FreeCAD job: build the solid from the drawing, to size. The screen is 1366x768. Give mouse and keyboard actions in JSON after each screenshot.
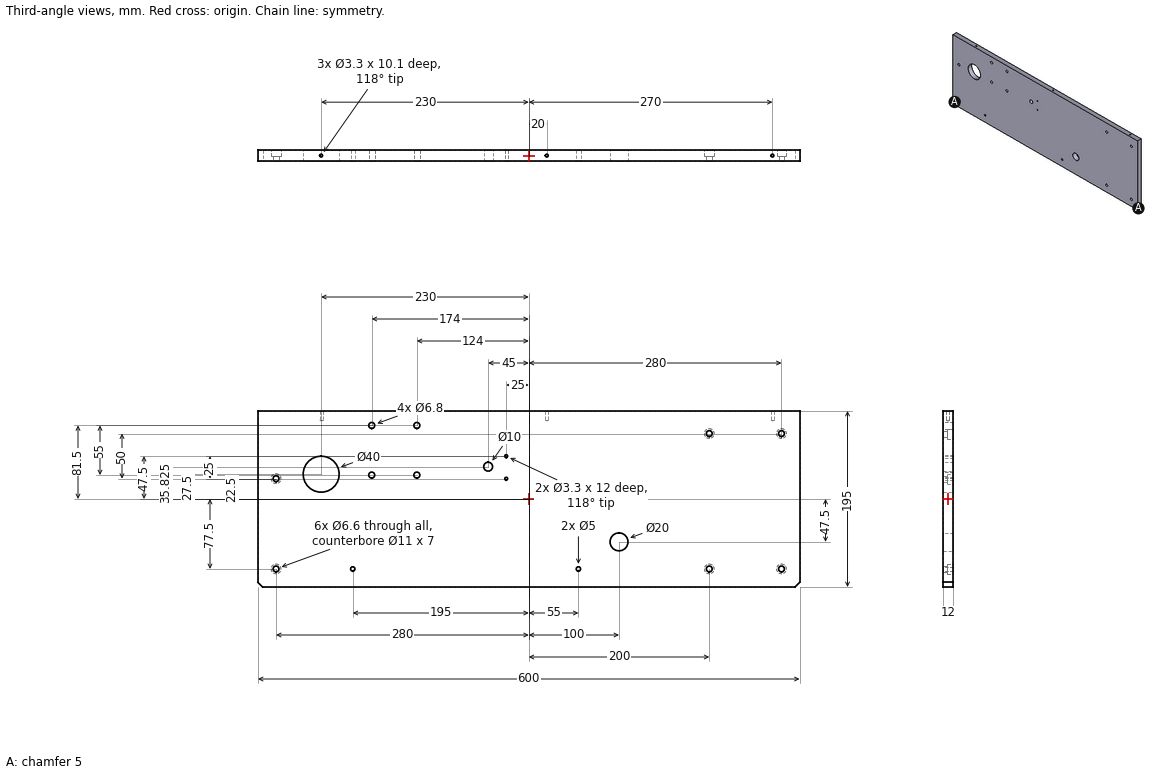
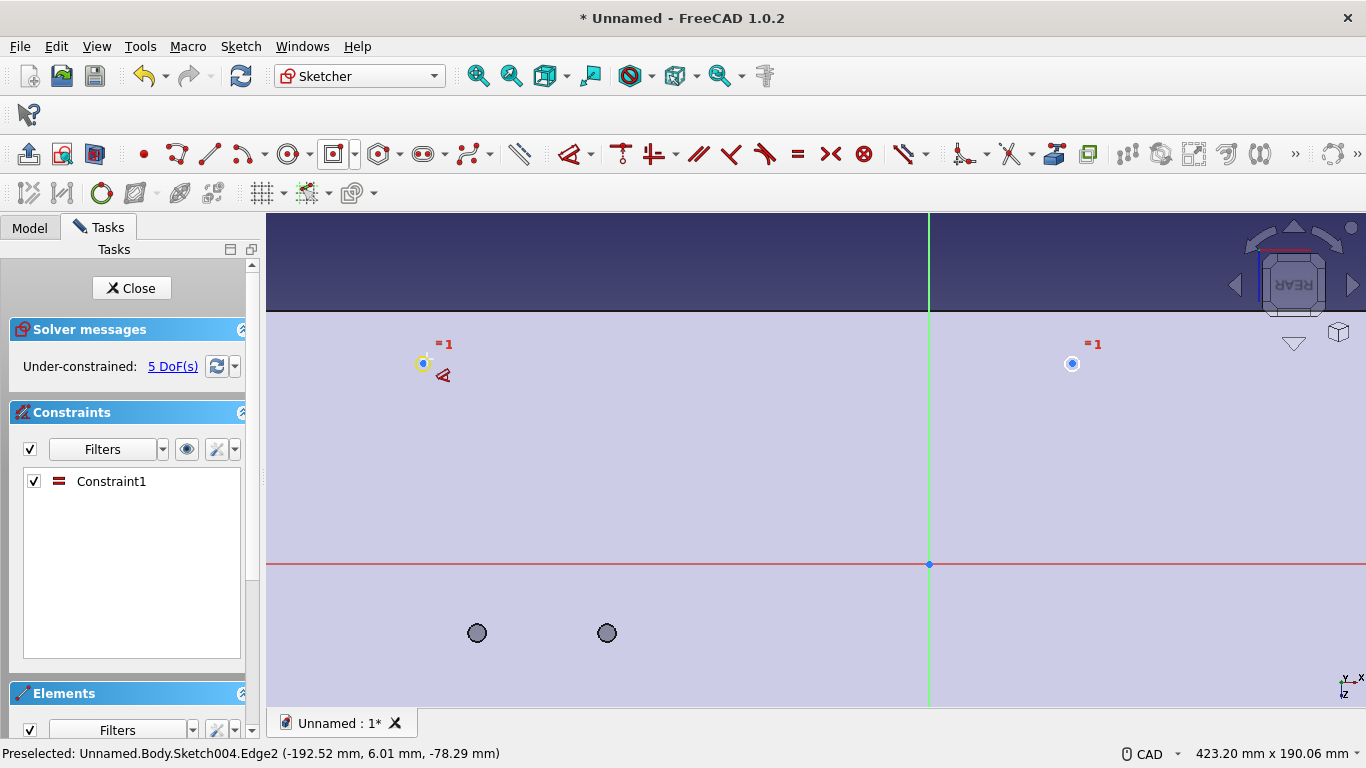
{"action": "scroll", "coordinate": [1077, 359], "scroll_direction": "up", "scroll_amount": 6}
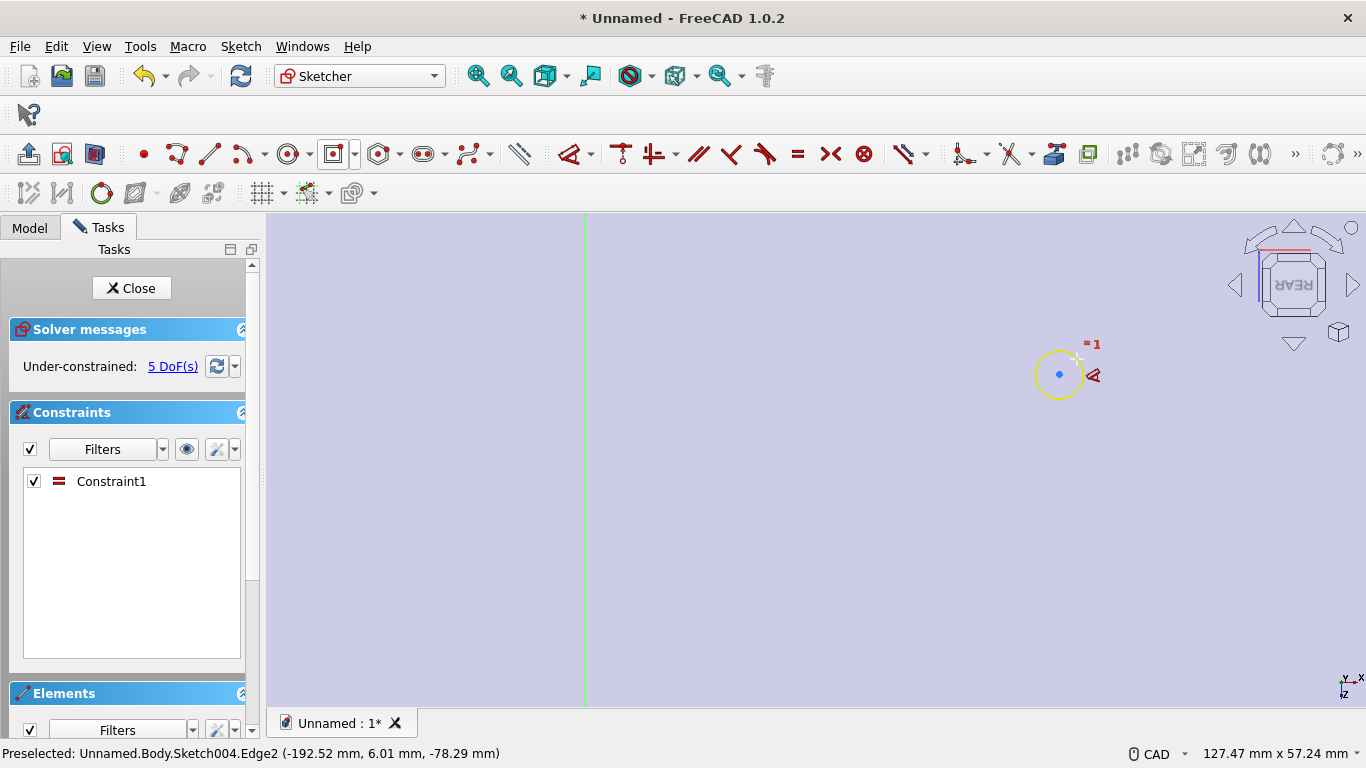
{"action": "left_click", "coordinate": [1076, 358]}
{"action": "left_click", "coordinate": [1098, 335]}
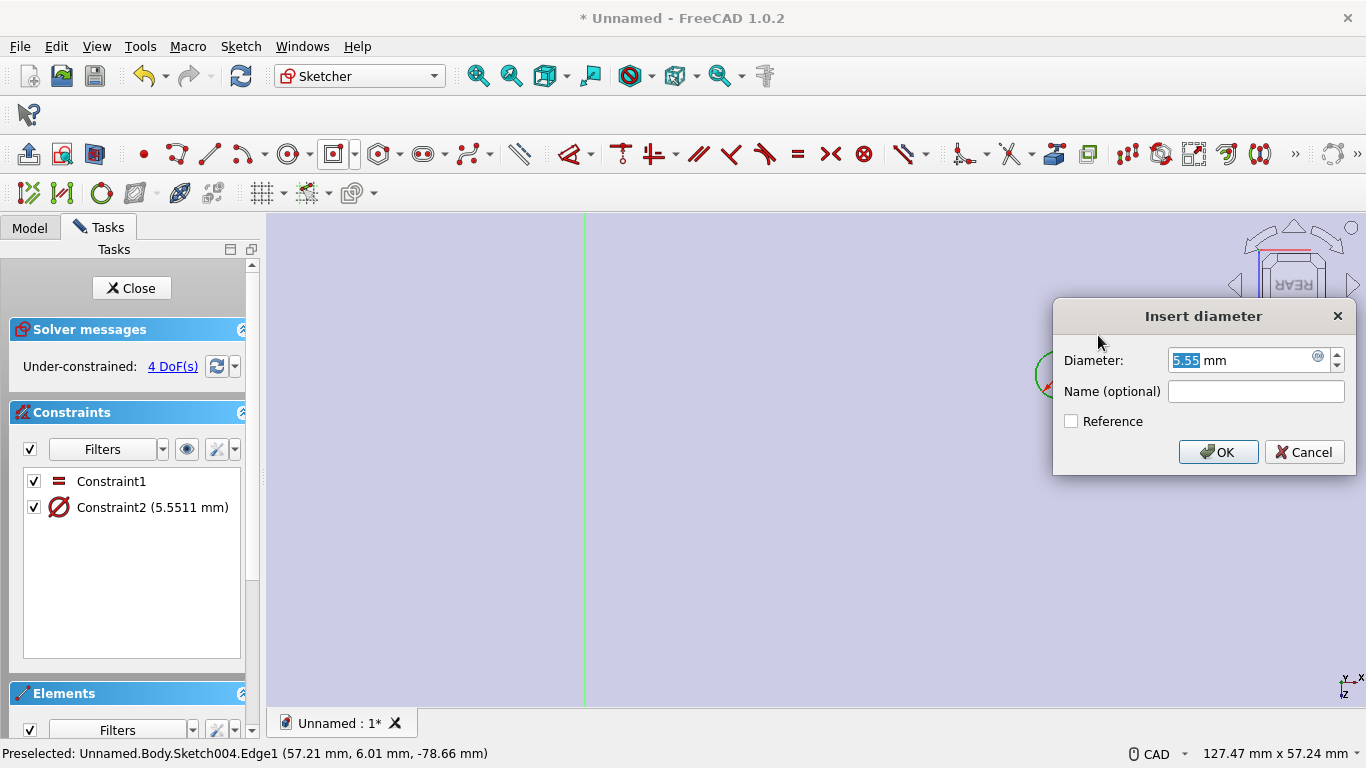
{"action": "type", "text": "5"}
{"action": "key", "text": "Return"}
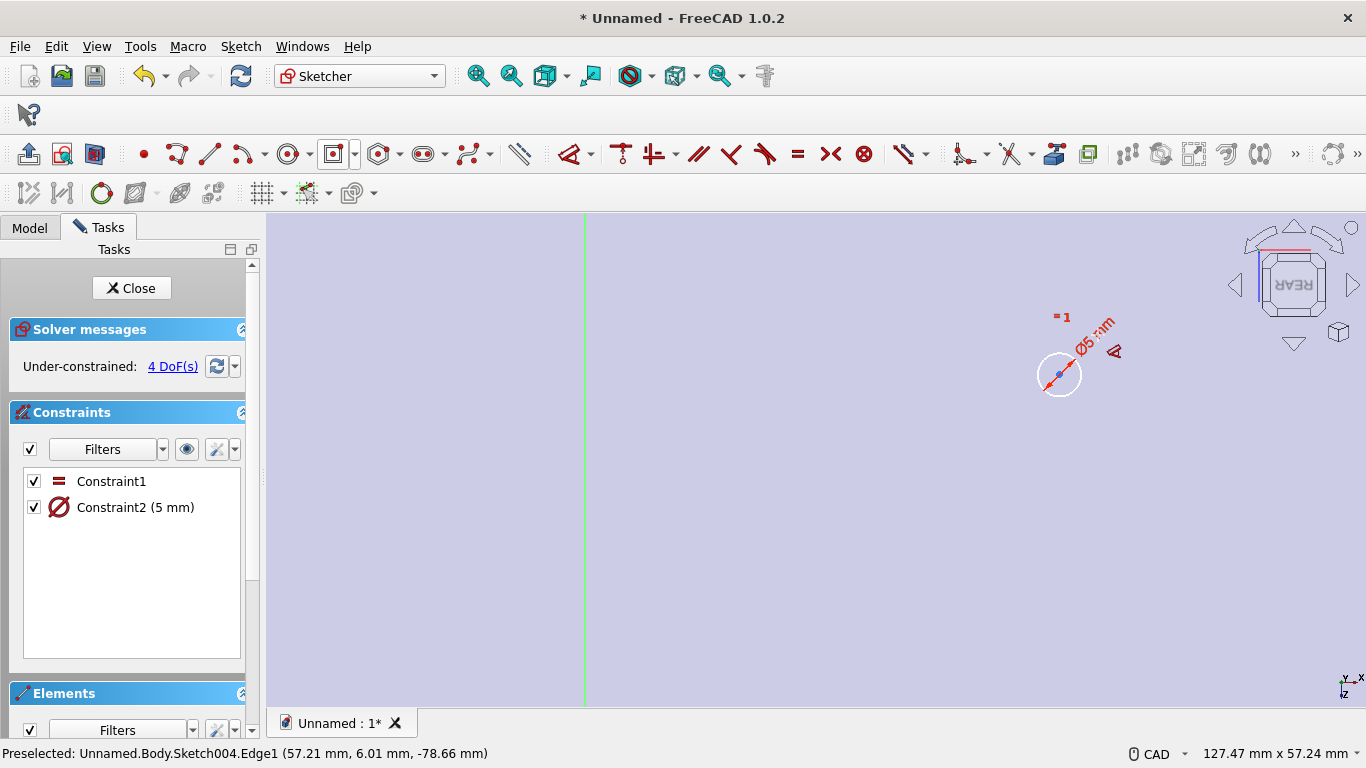
{"action": "left_click", "coordinate": [1060, 375]}
{"action": "left_click", "coordinate": [822, 341]}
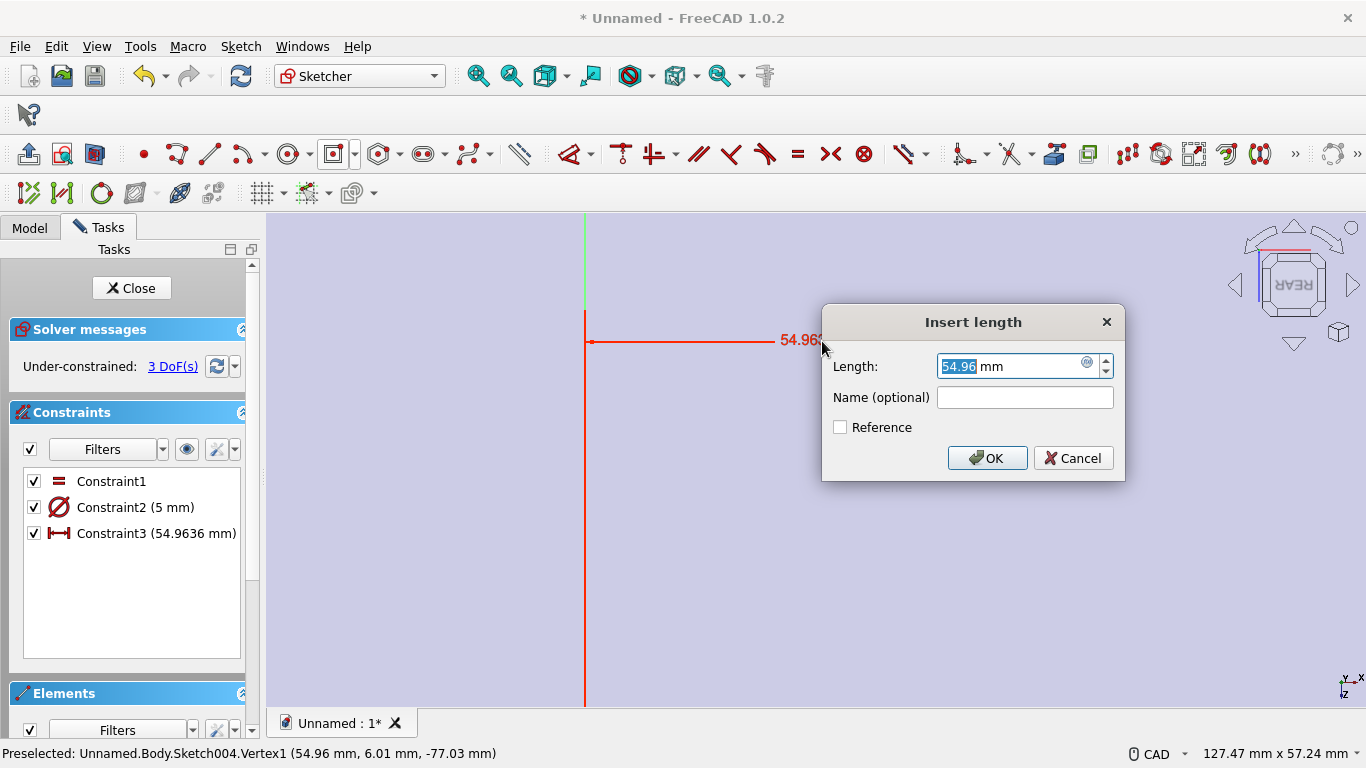
{"action": "type", "text": "55"}
{"action": "key", "text": "Return"}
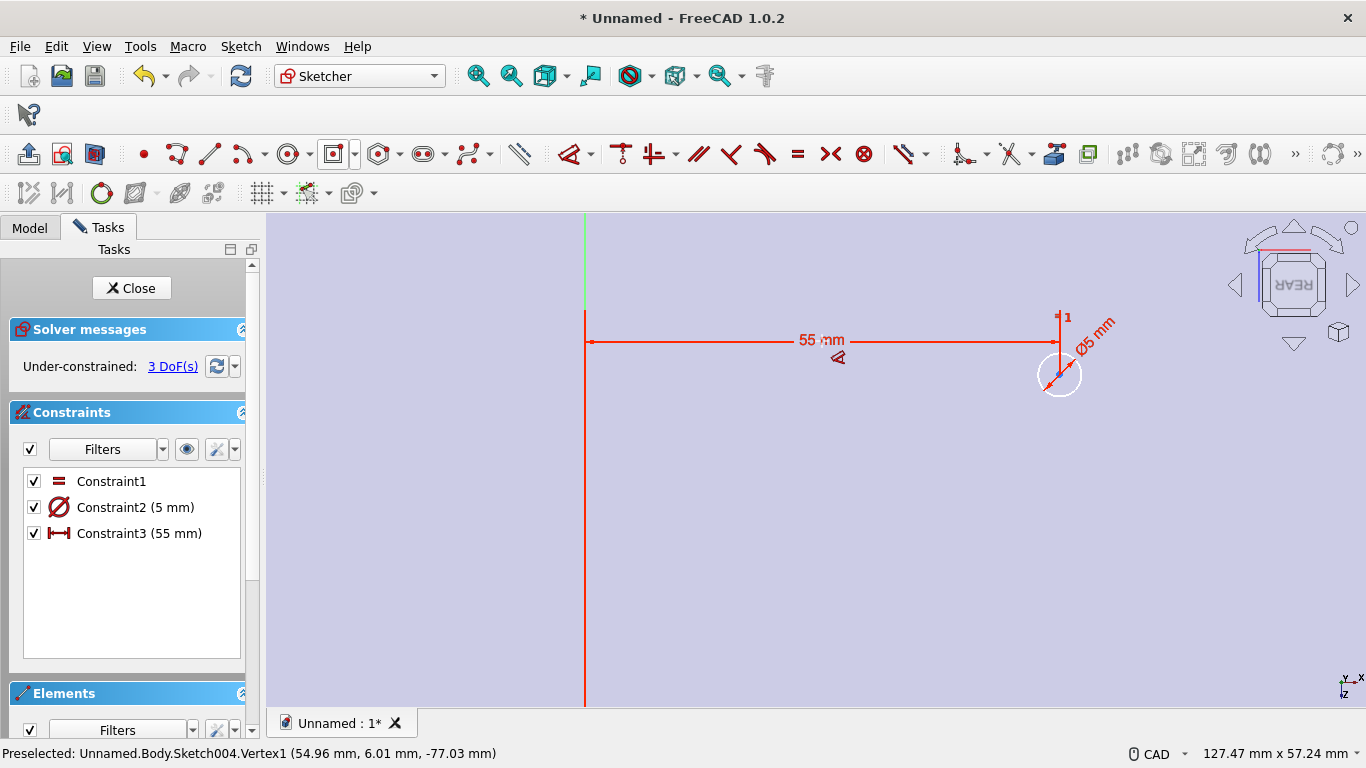
{"action": "scroll", "coordinate": [1078, 359], "scroll_direction": "down", "scroll_amount": 6}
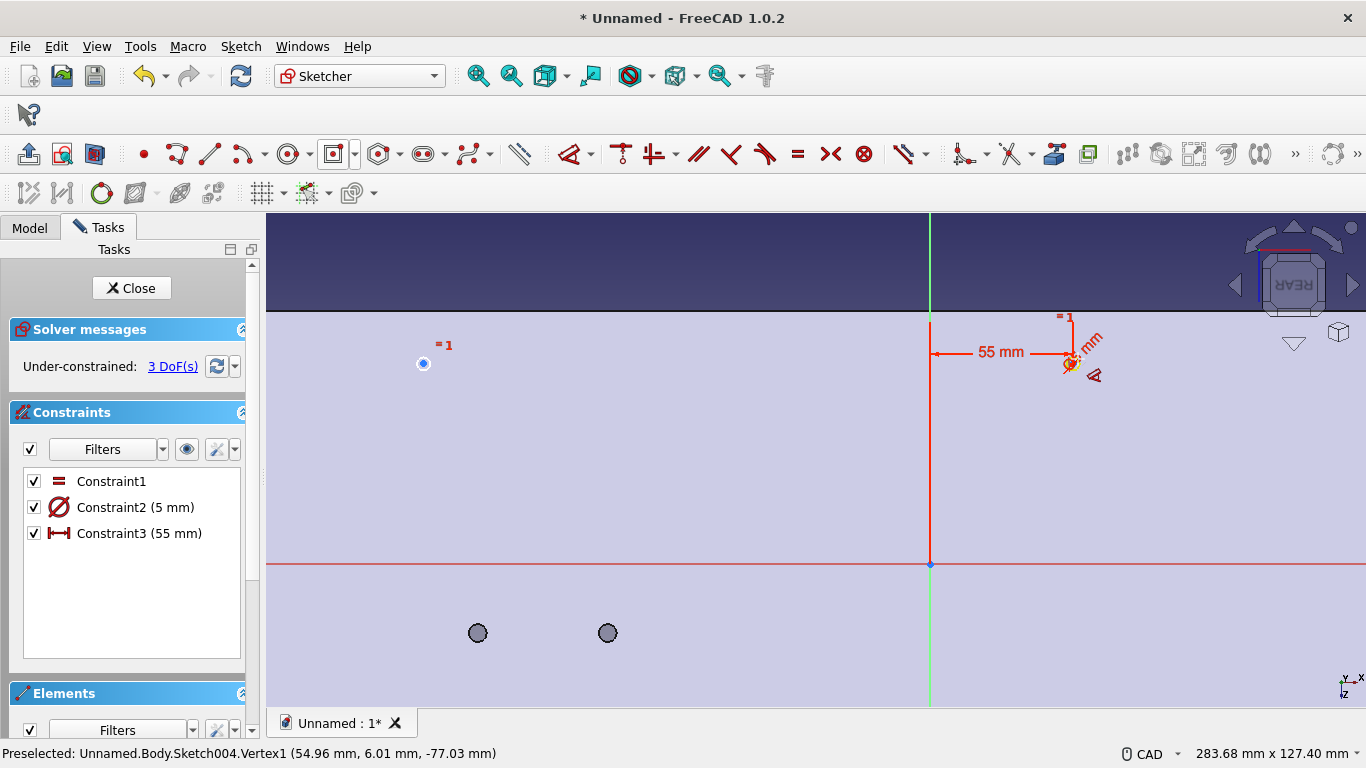
{"action": "left_click", "coordinate": [424, 364]}
{"action": "left_click", "coordinate": [677, 598]}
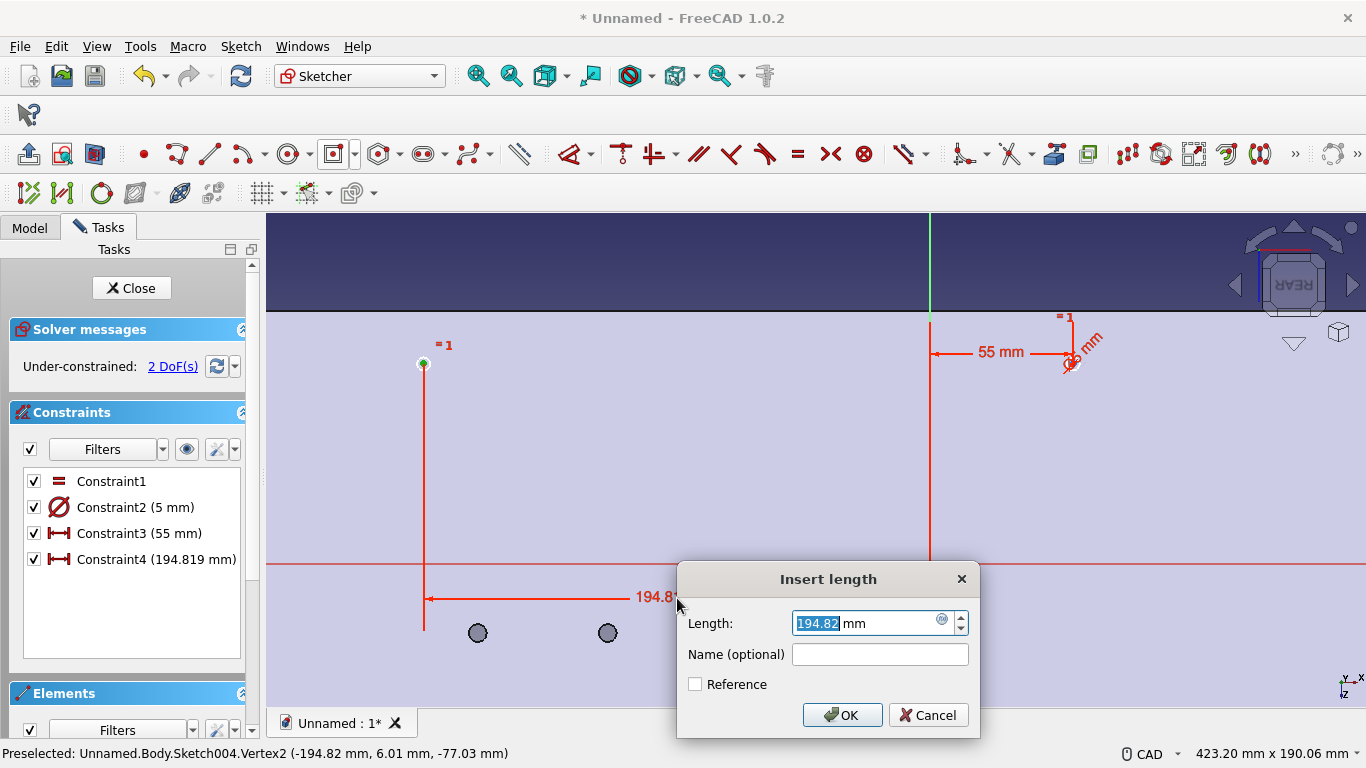
{"action": "type", "text": "195"}
{"action": "key", "text": "Return"}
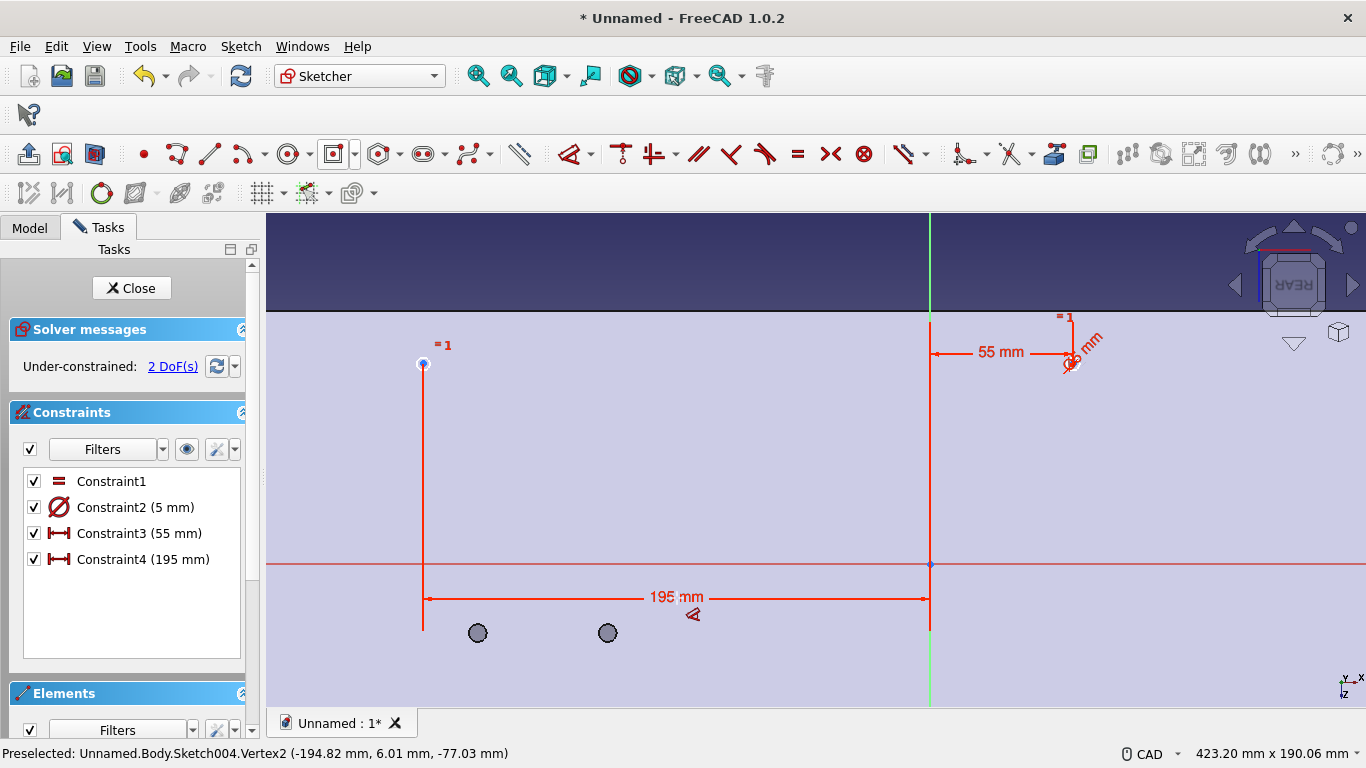
{"action": "left_click", "coordinate": [1073, 364]}
{"action": "left_click", "coordinate": [1107, 464]}